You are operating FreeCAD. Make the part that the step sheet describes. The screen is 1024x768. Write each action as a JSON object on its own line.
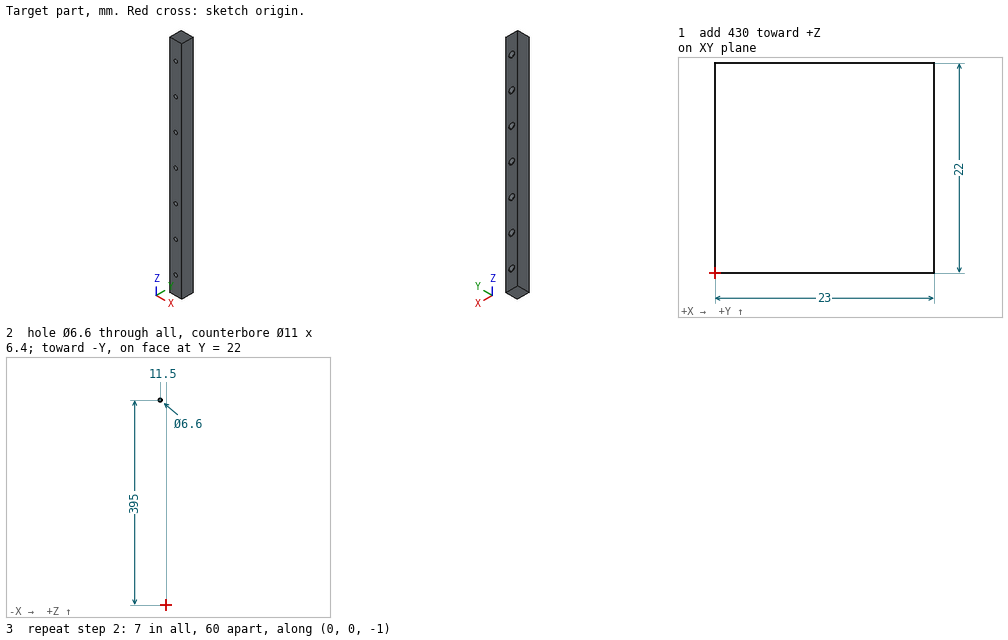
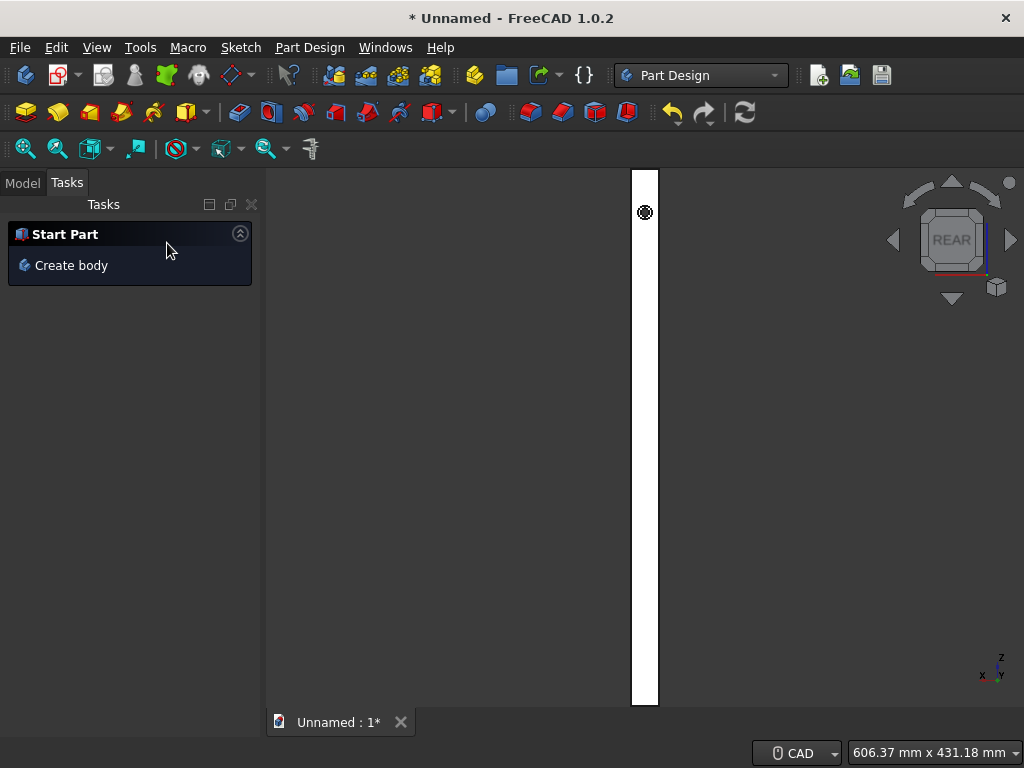
{"action": "left_click", "coordinate": [23, 182]}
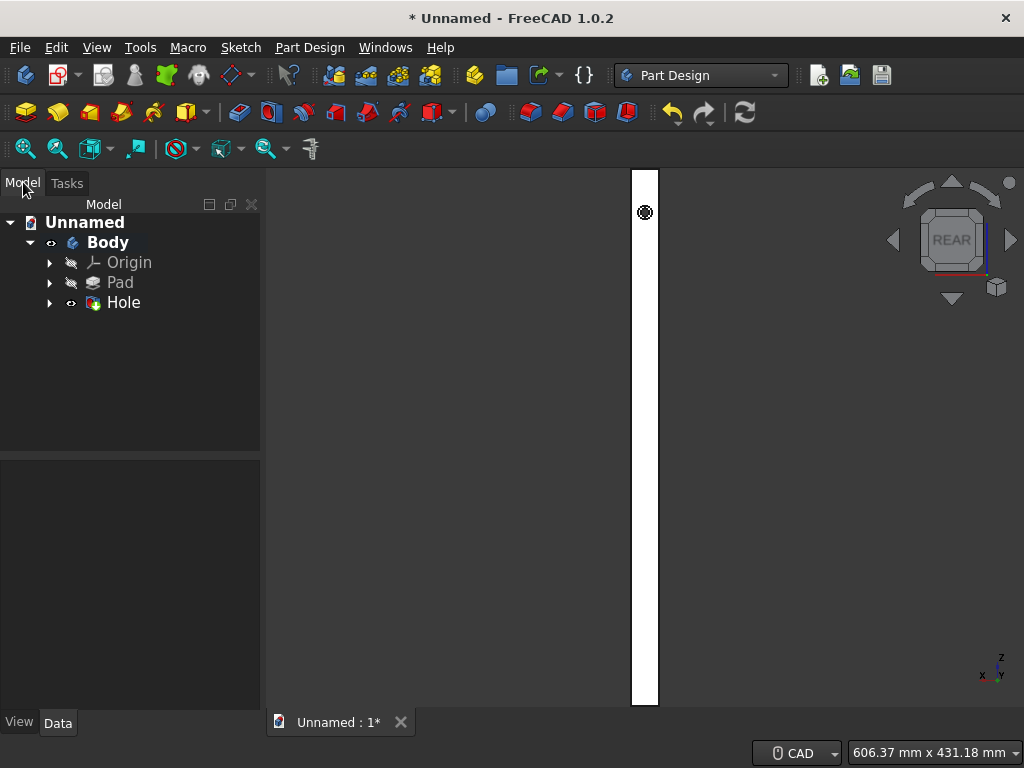
{"action": "left_click", "coordinate": [116, 303]}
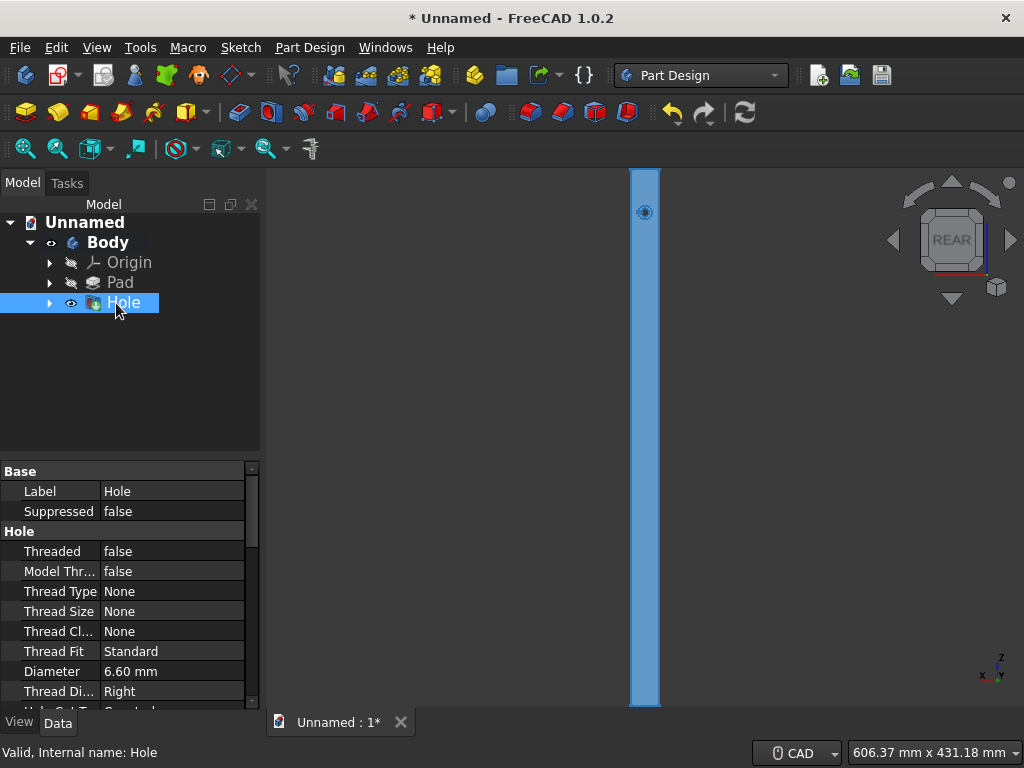
{"action": "left_click", "coordinate": [366, 76]}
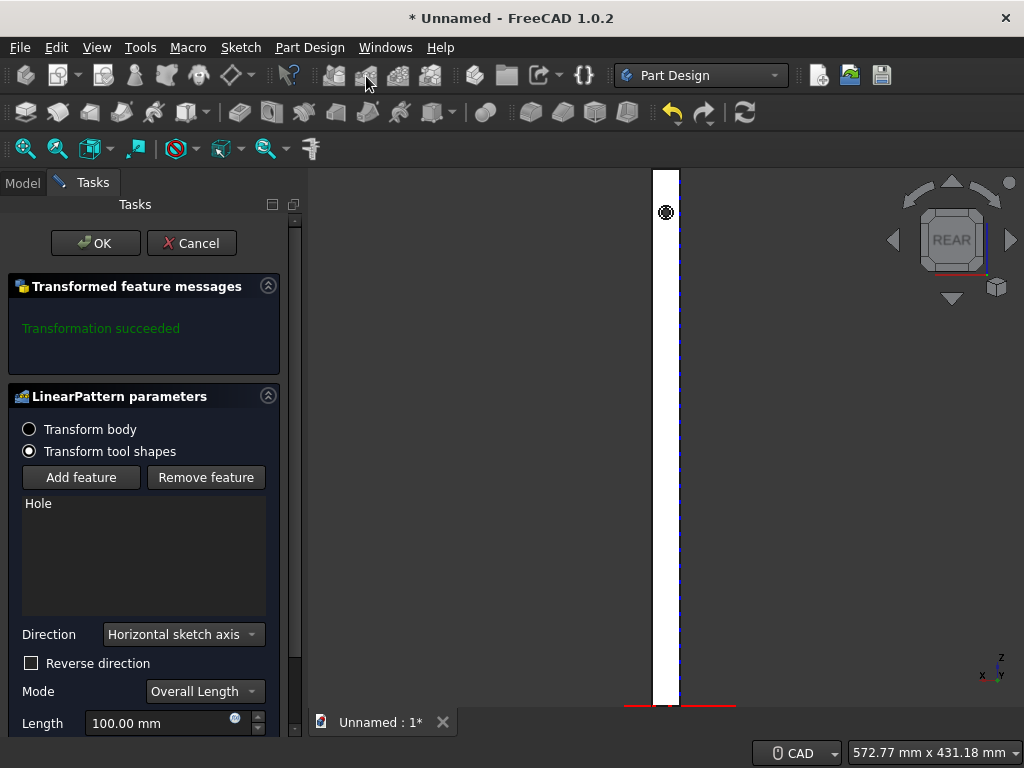
{"action": "left_click", "coordinate": [184, 634]}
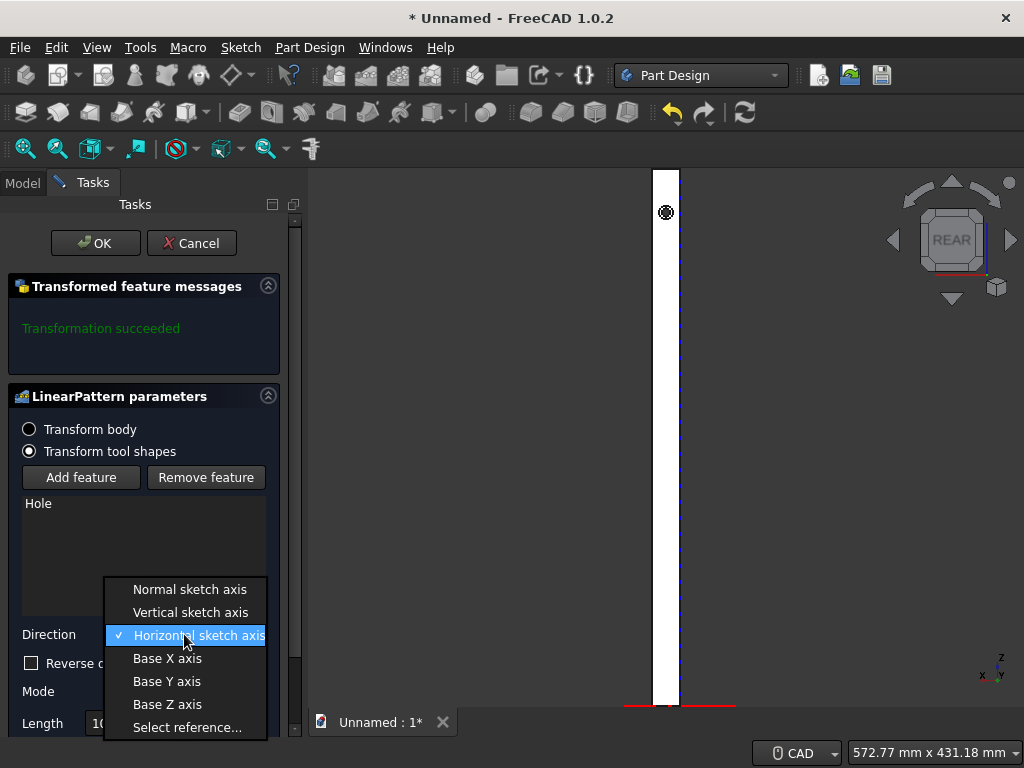
{"action": "left_click", "coordinate": [184, 704]}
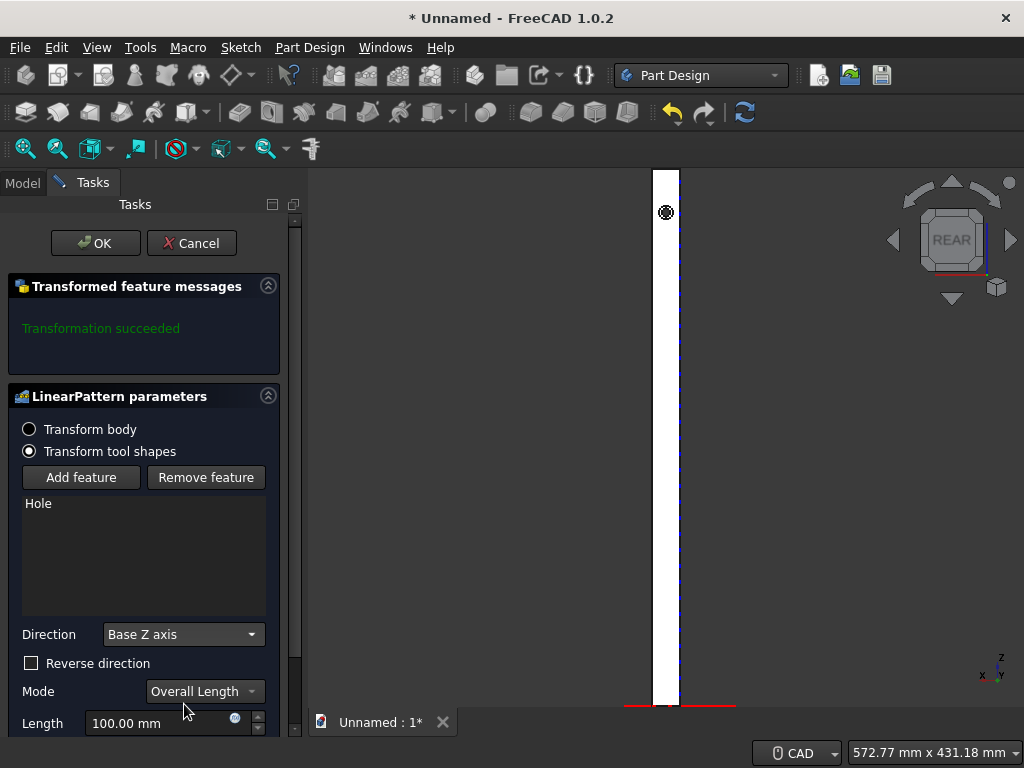
{"action": "left_click", "coordinate": [206, 692]}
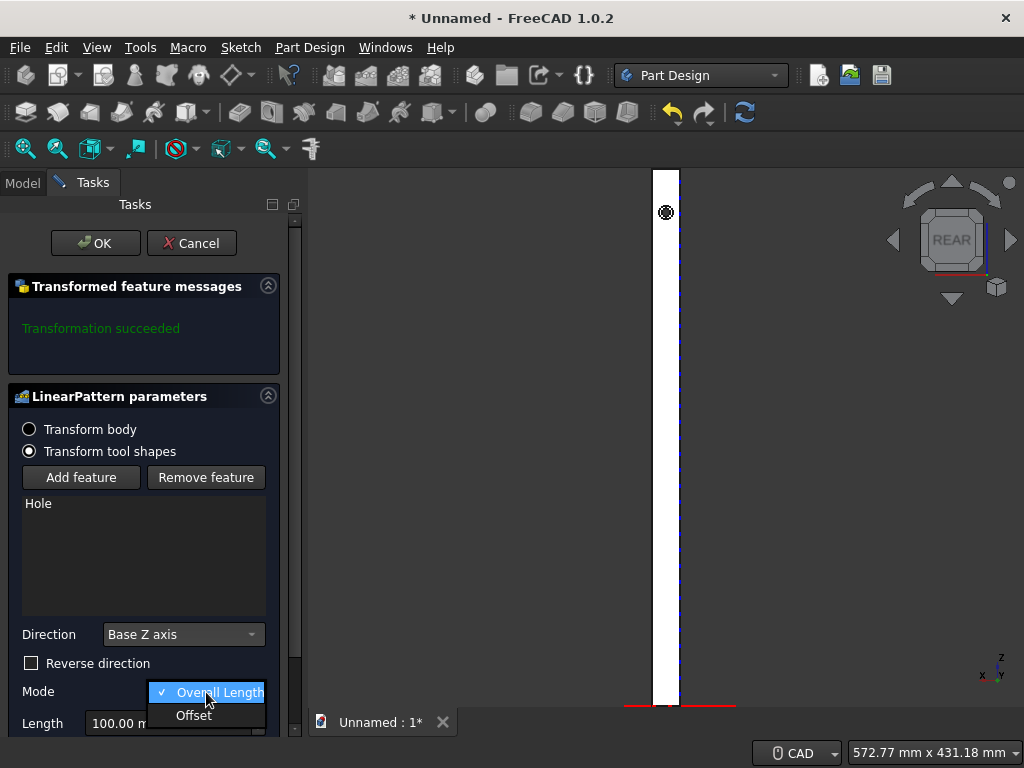
{"action": "left_click", "coordinate": [206, 716]}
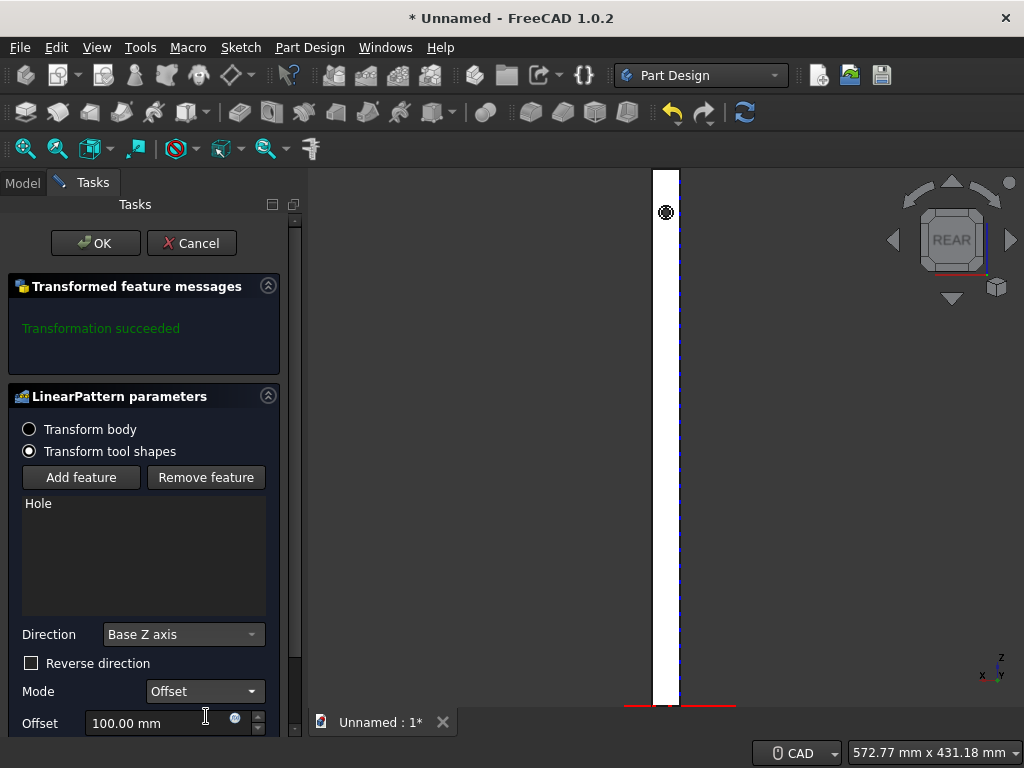
{"action": "triple_click", "coordinate": [168, 723]}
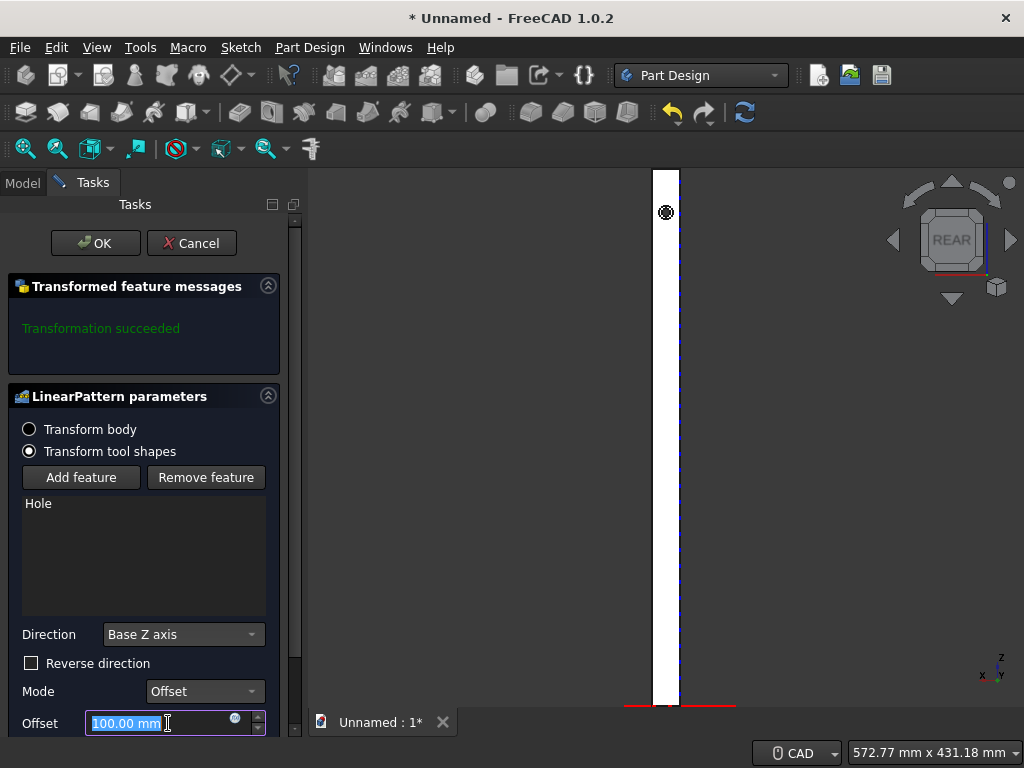
{"action": "type", "text": "60"}
{"action": "key", "text": "Tab"}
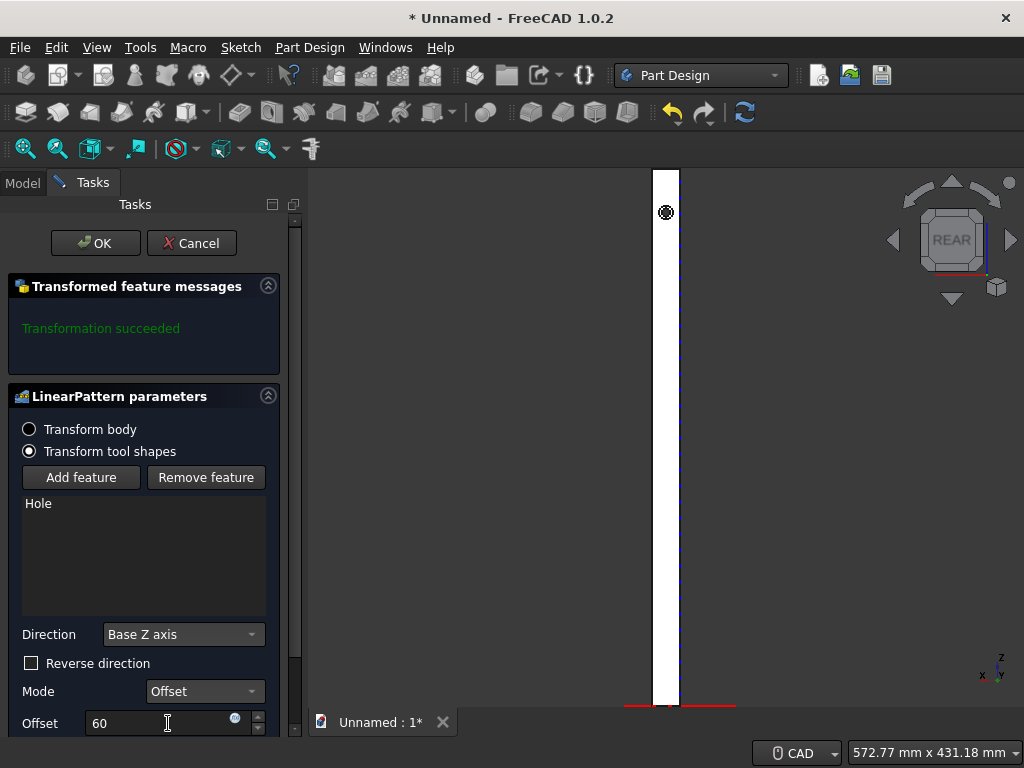
{"action": "scroll", "coordinate": [295, 475], "scroll_direction": "down", "scroll_amount": 2}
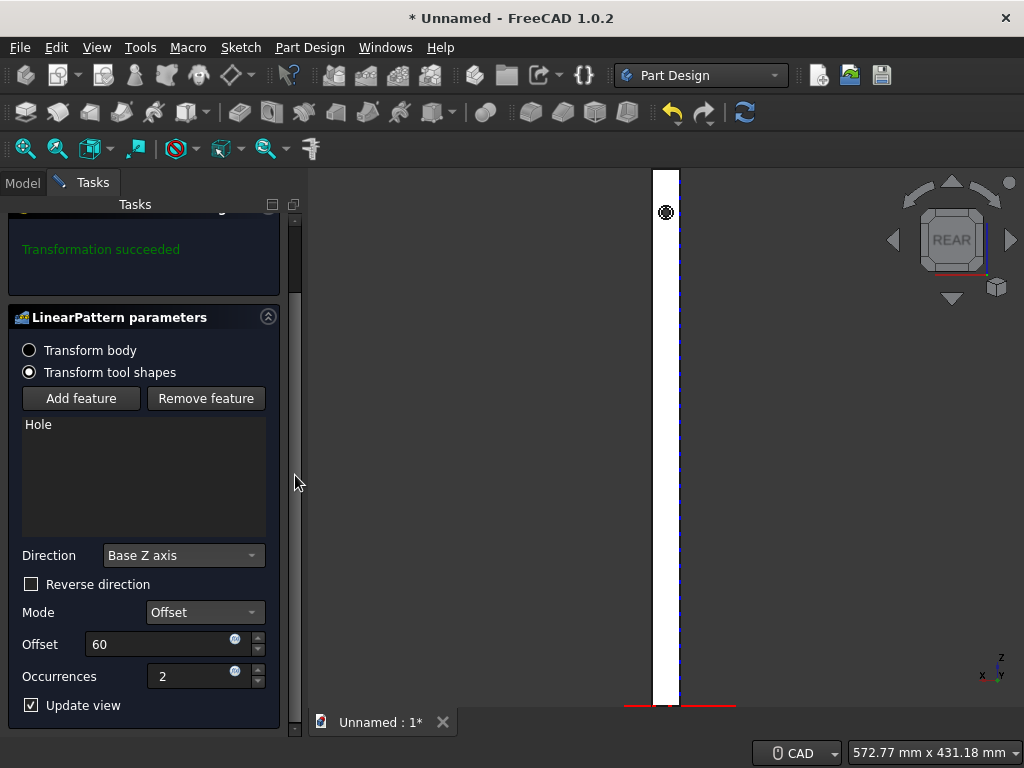
{"action": "triple_click", "coordinate": [198, 676]}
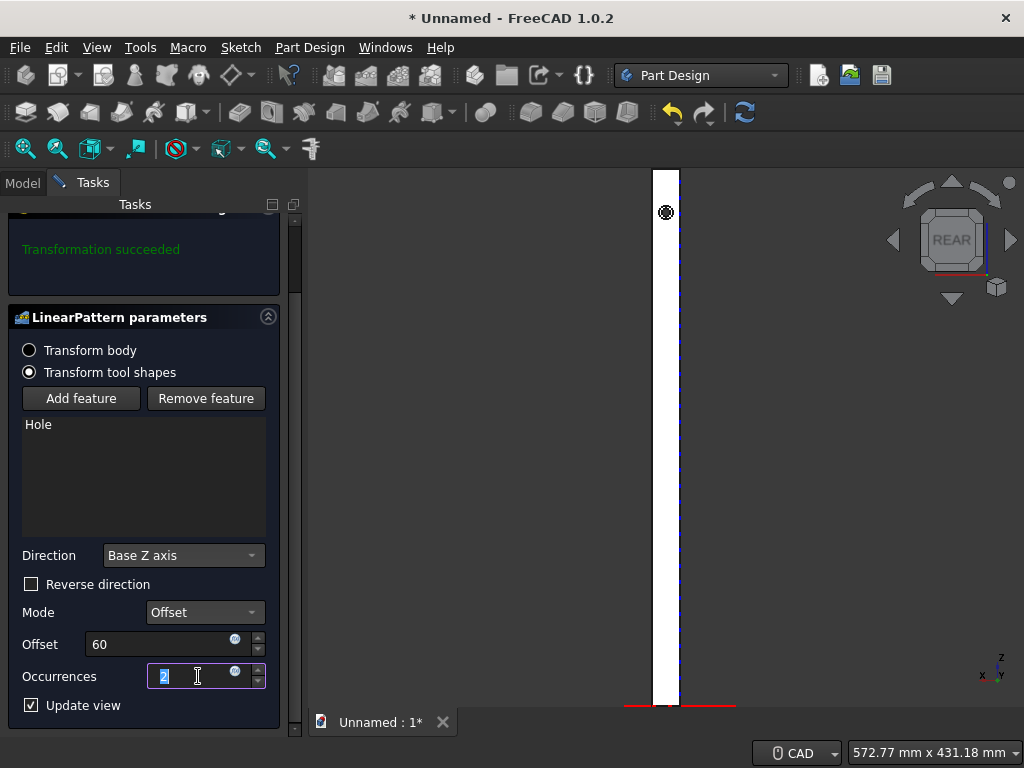
{"action": "type", "text": "7"}
{"action": "key", "text": "Tab"}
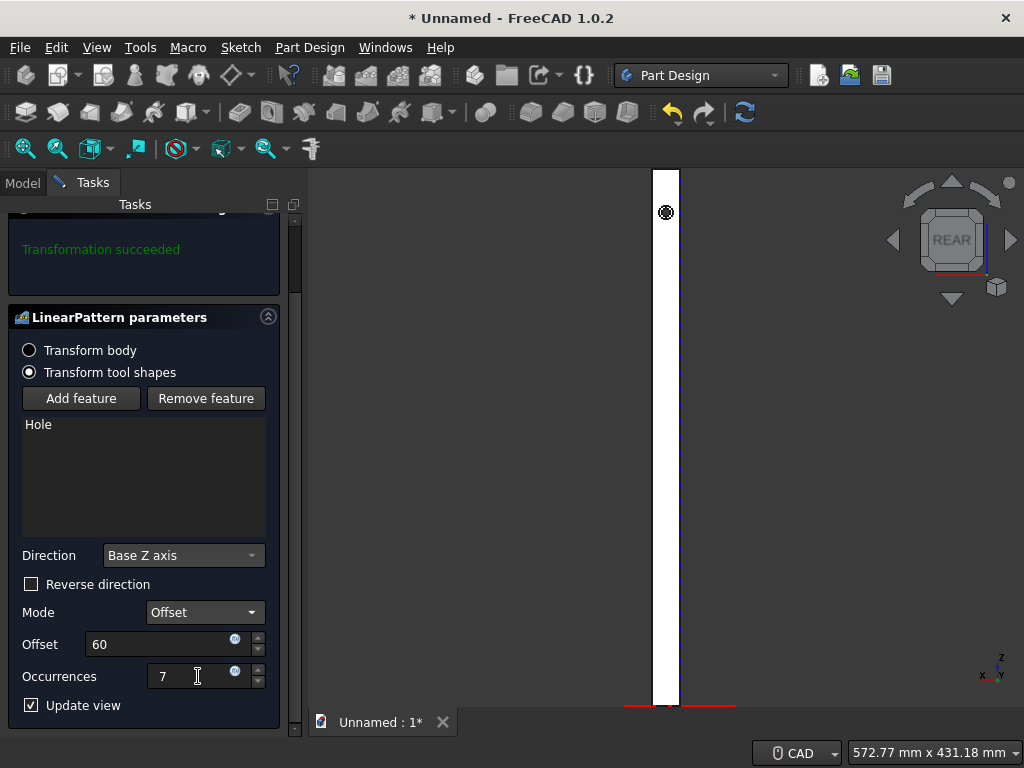
{"action": "left_click", "coordinate": [30, 584]}